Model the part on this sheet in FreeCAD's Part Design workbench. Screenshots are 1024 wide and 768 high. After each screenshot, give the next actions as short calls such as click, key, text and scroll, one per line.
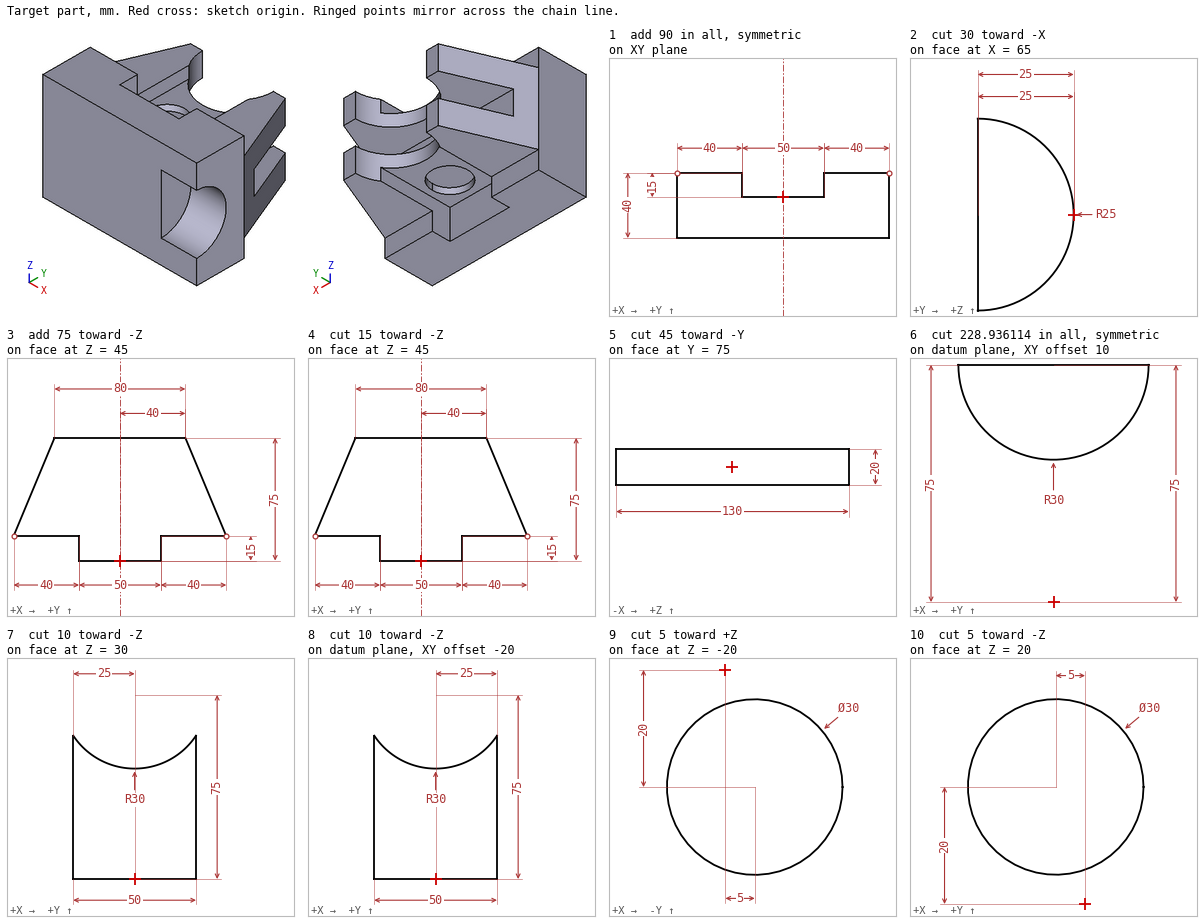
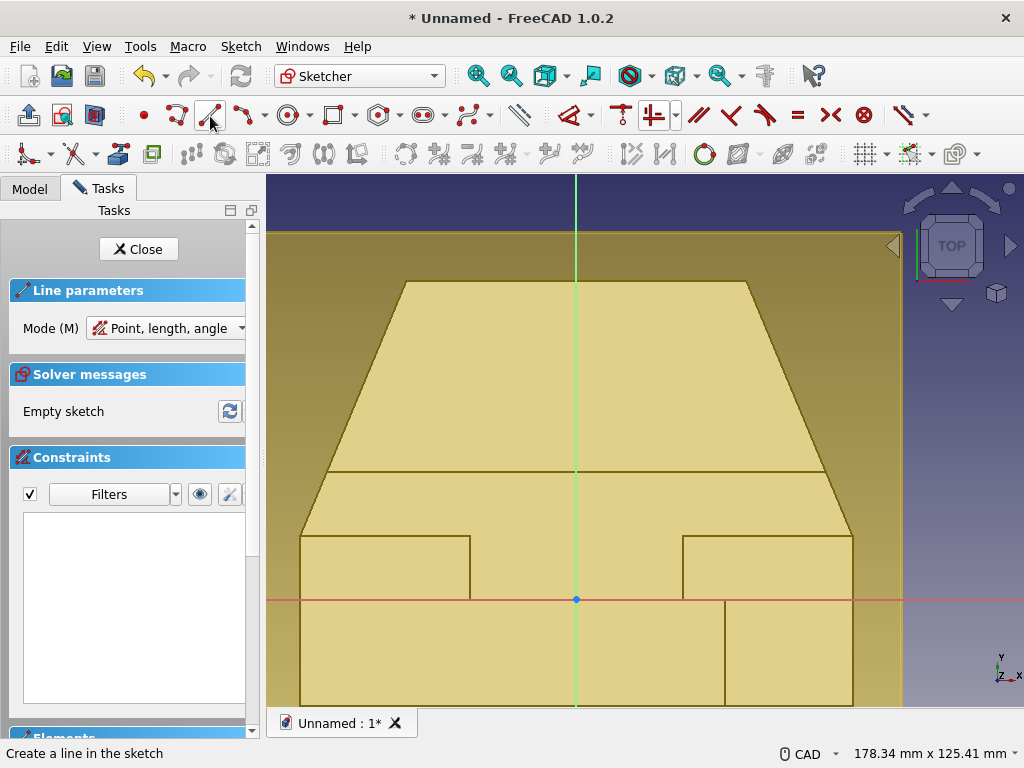
click(449, 281)
click(704, 281)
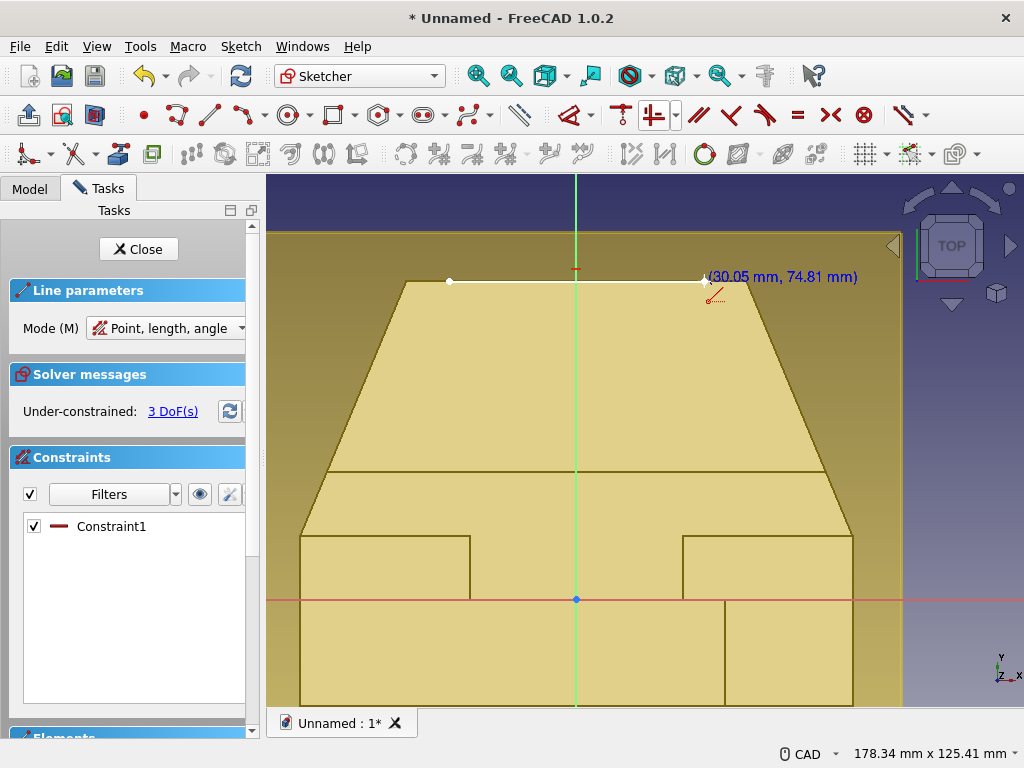
click(242, 116)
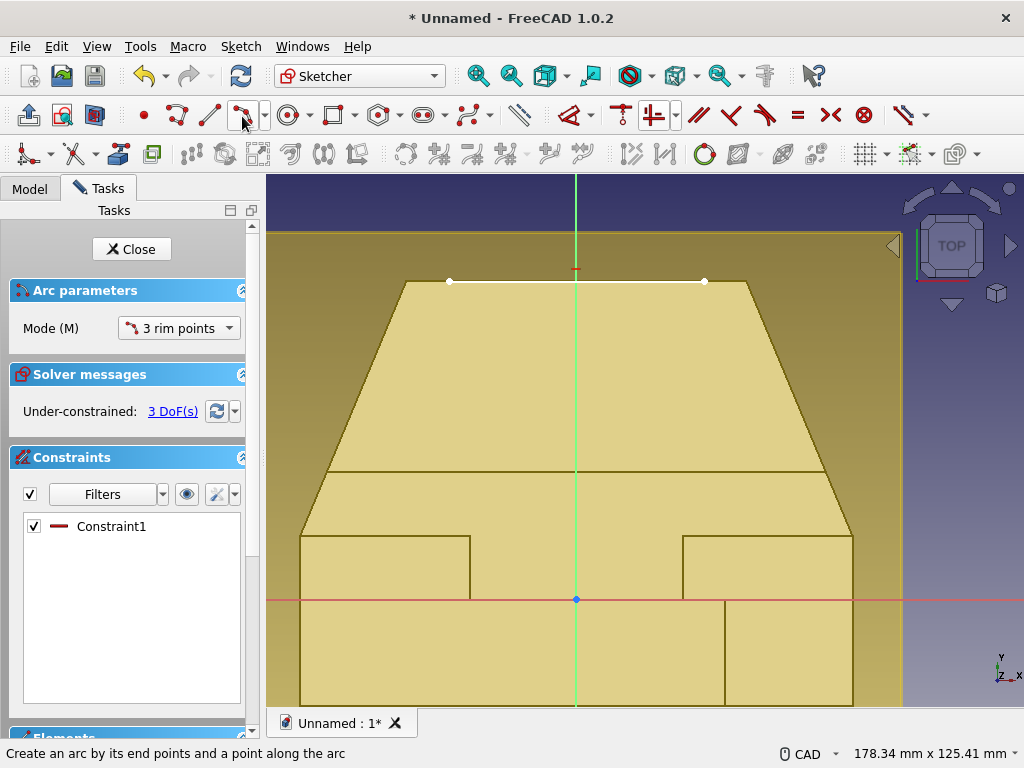
click(704, 282)
click(449, 282)
click(537, 402)
key(Escape)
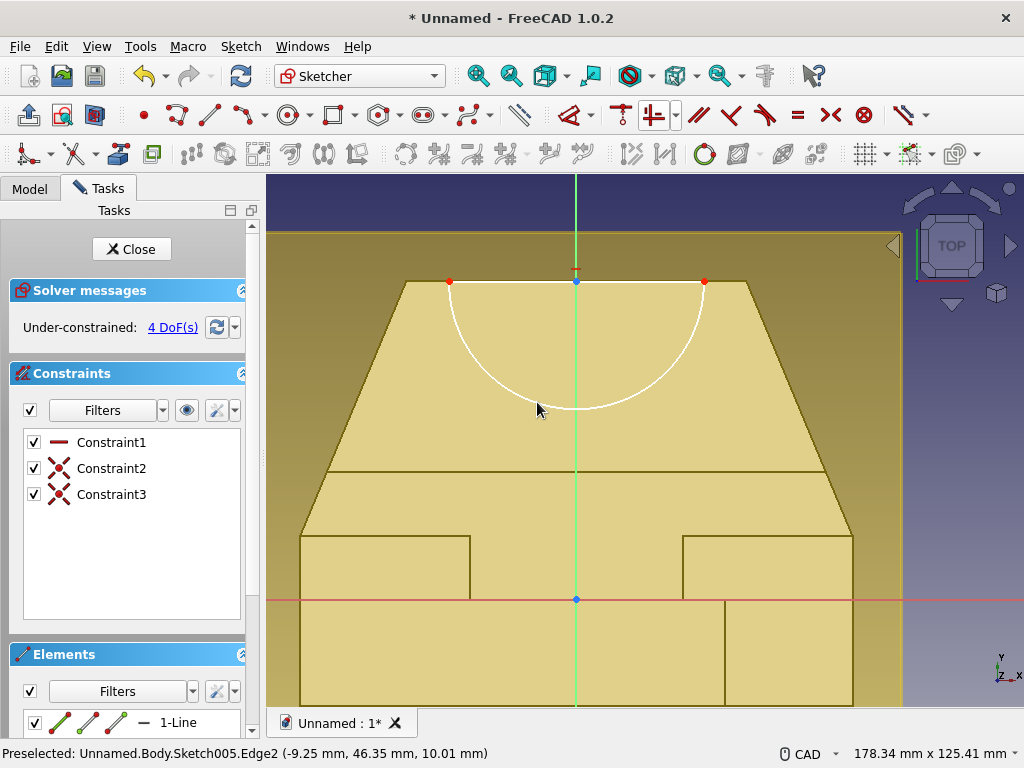
click(576, 282)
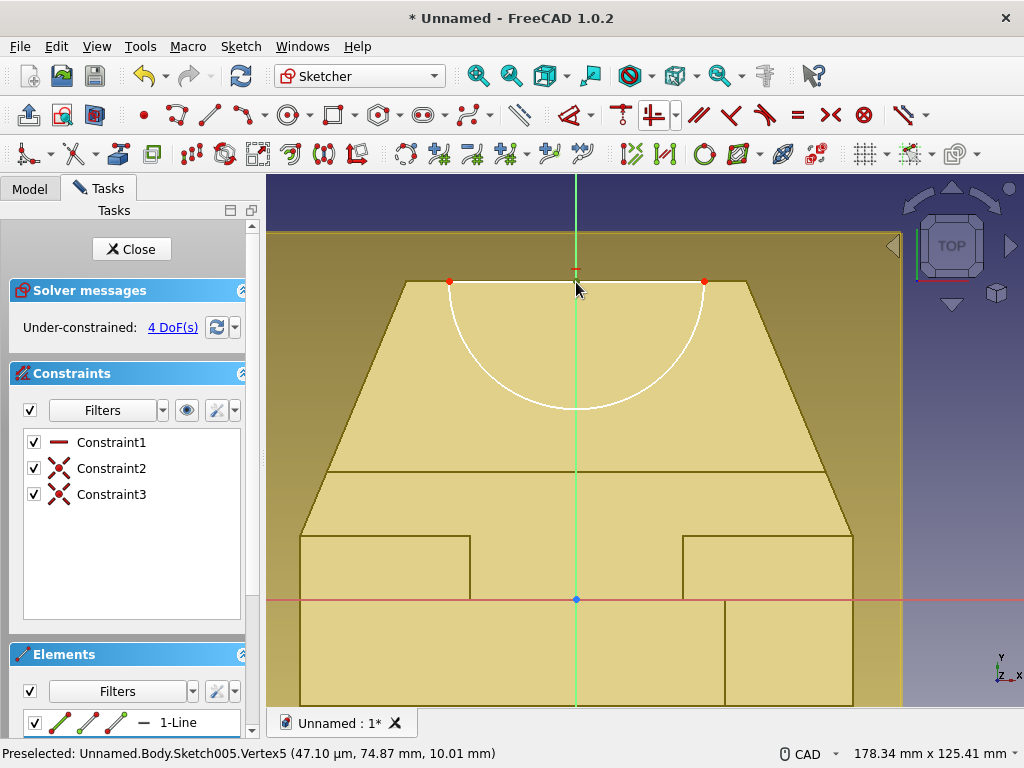
click(576, 645)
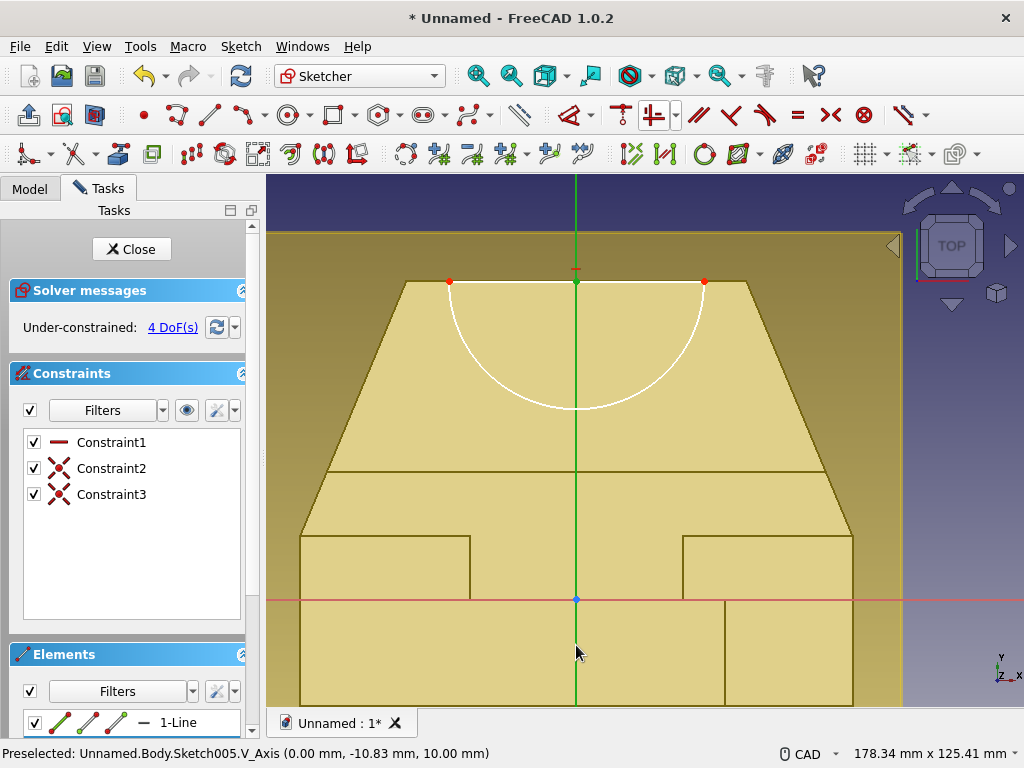
key(c)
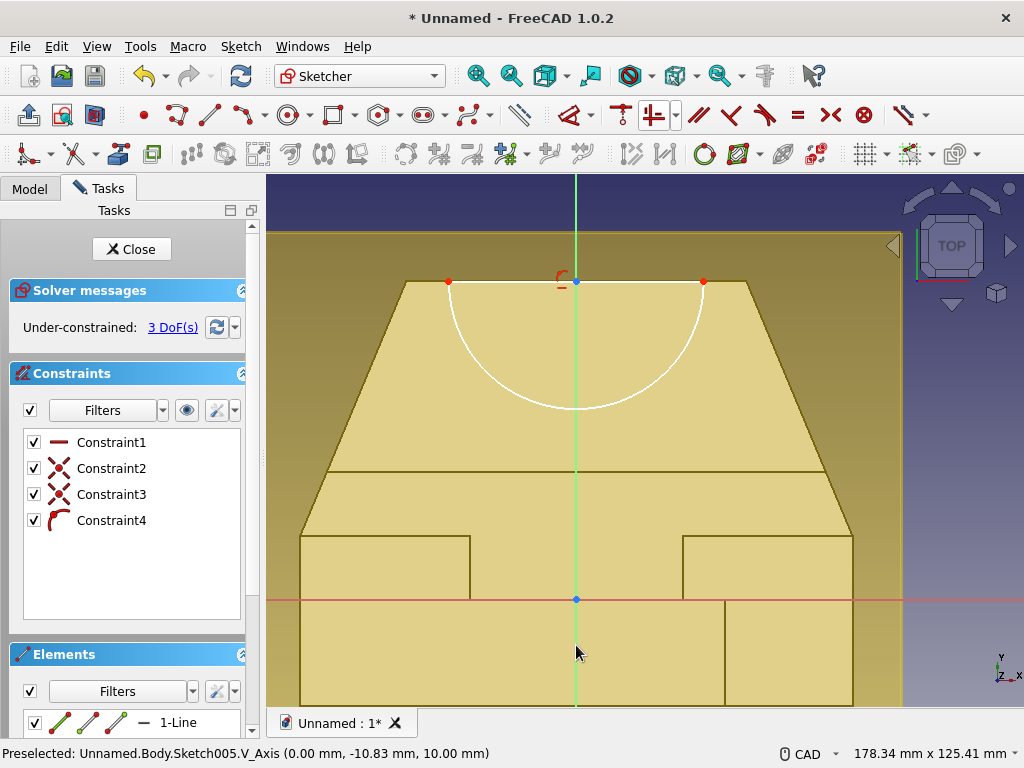
key(d)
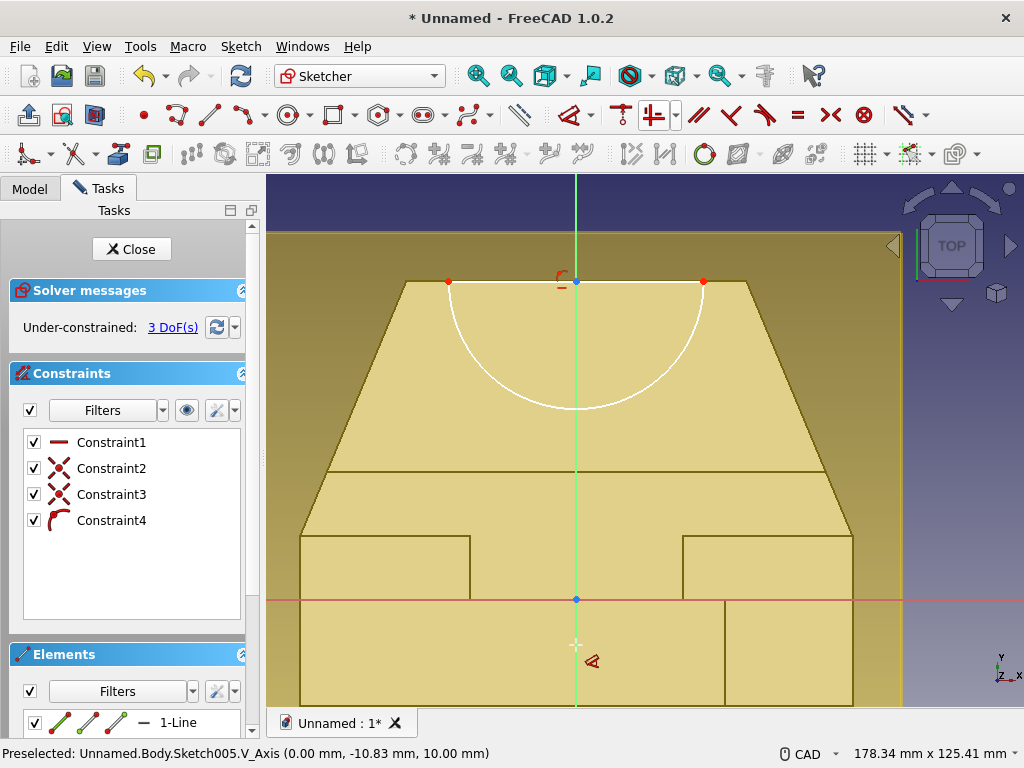
click(502, 385)
click(483, 411)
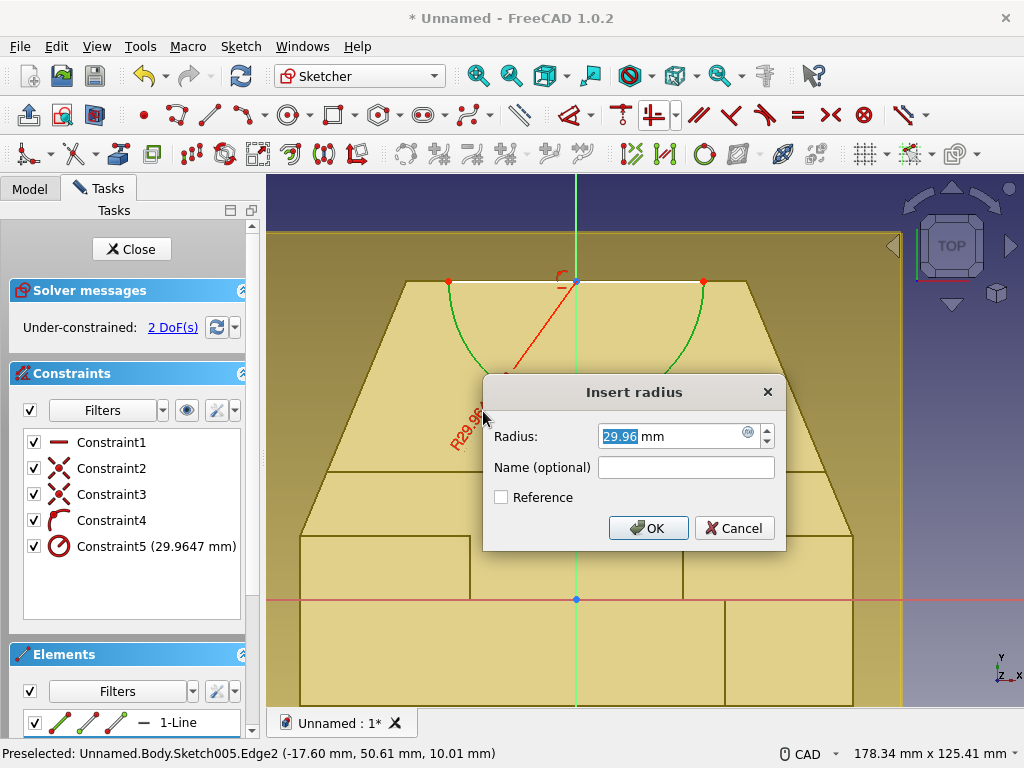
text(30)
key(Return)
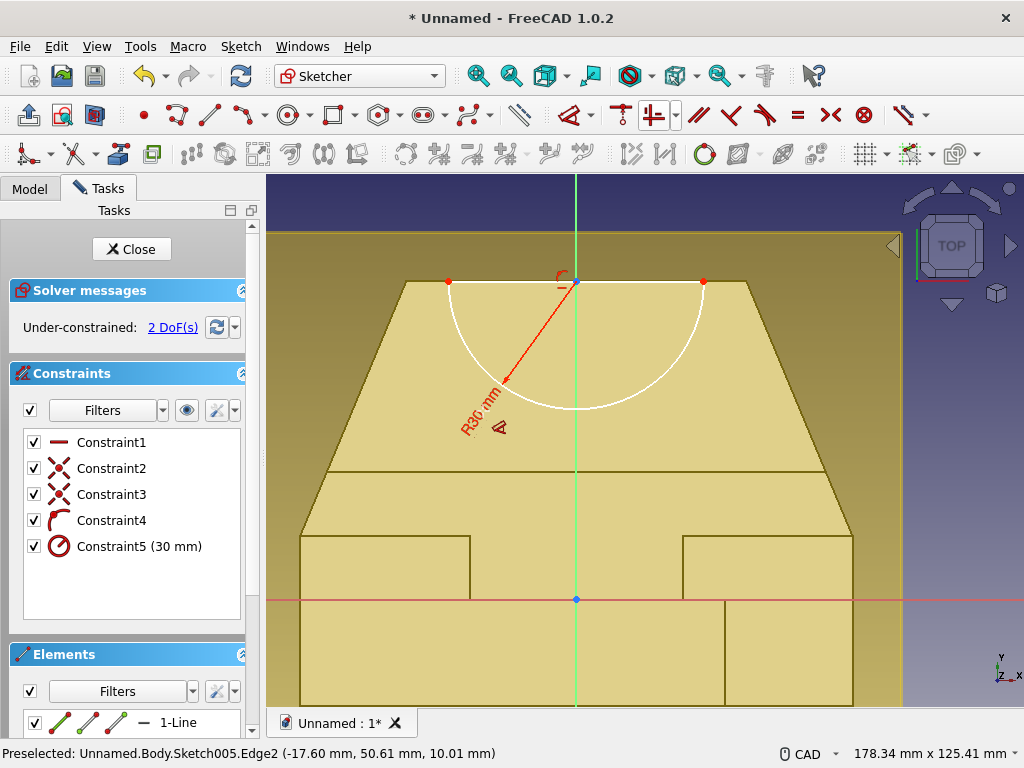
click(449, 282)
click(415, 441)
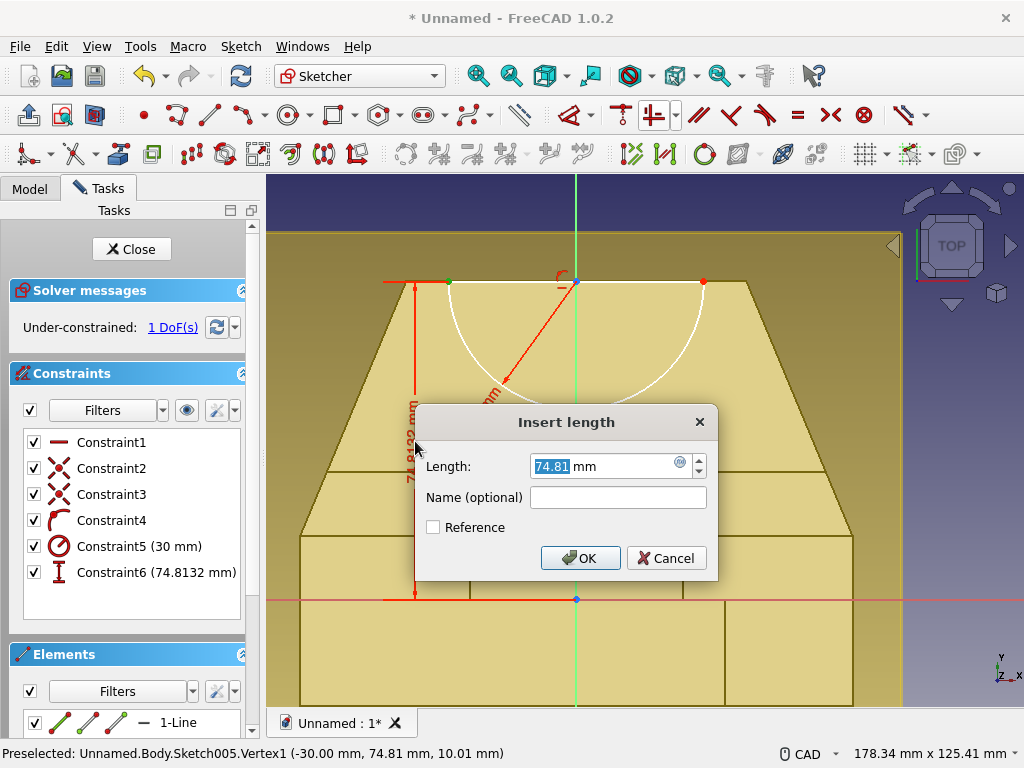
text(75)
key(Return)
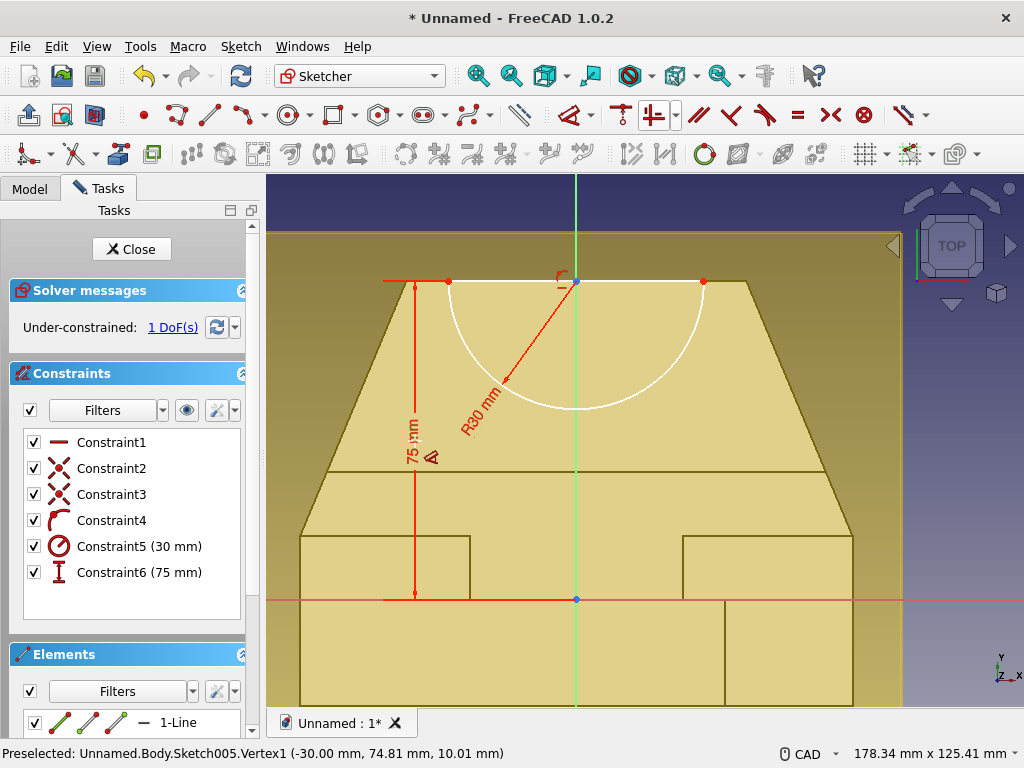
click(576, 282)
click(610, 441)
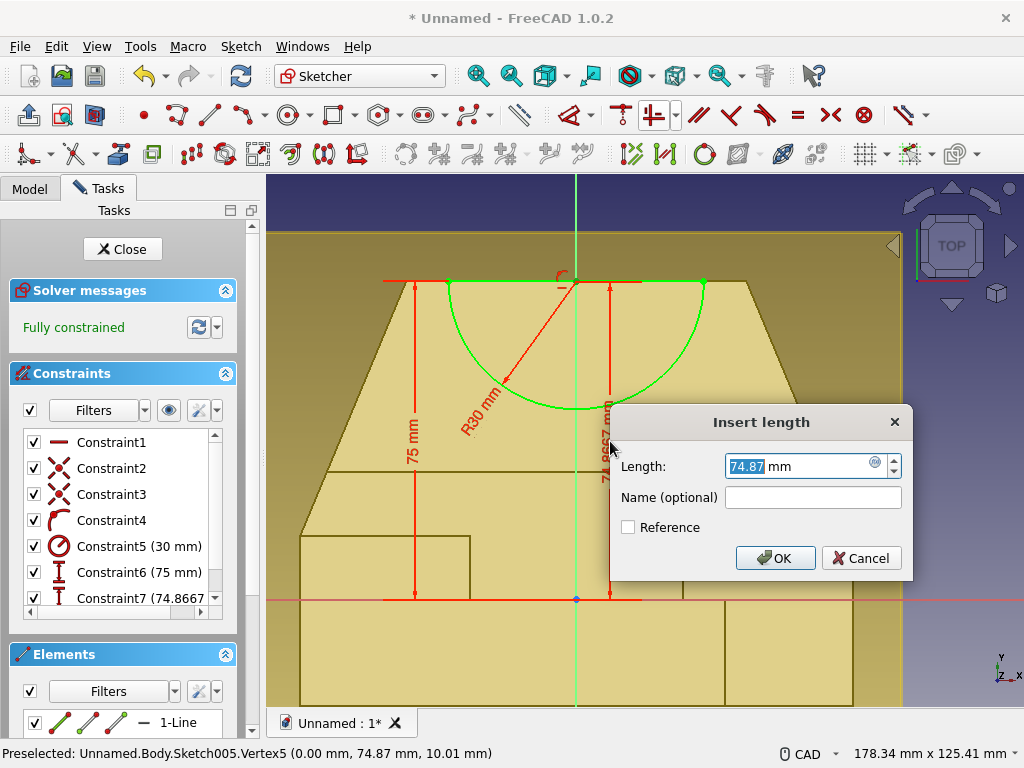
text(75)
key(Return)
key(Escape)